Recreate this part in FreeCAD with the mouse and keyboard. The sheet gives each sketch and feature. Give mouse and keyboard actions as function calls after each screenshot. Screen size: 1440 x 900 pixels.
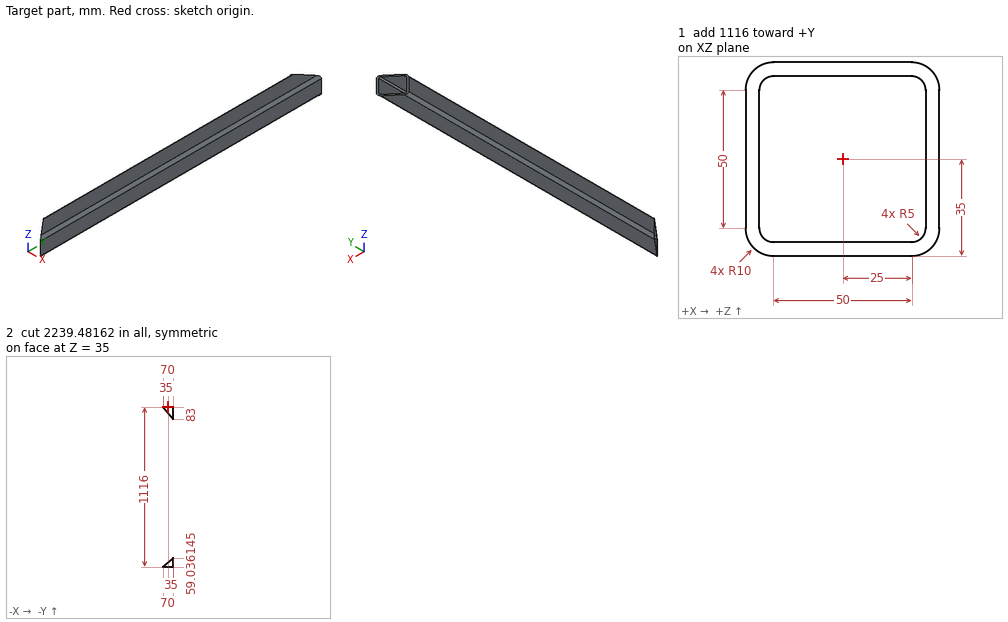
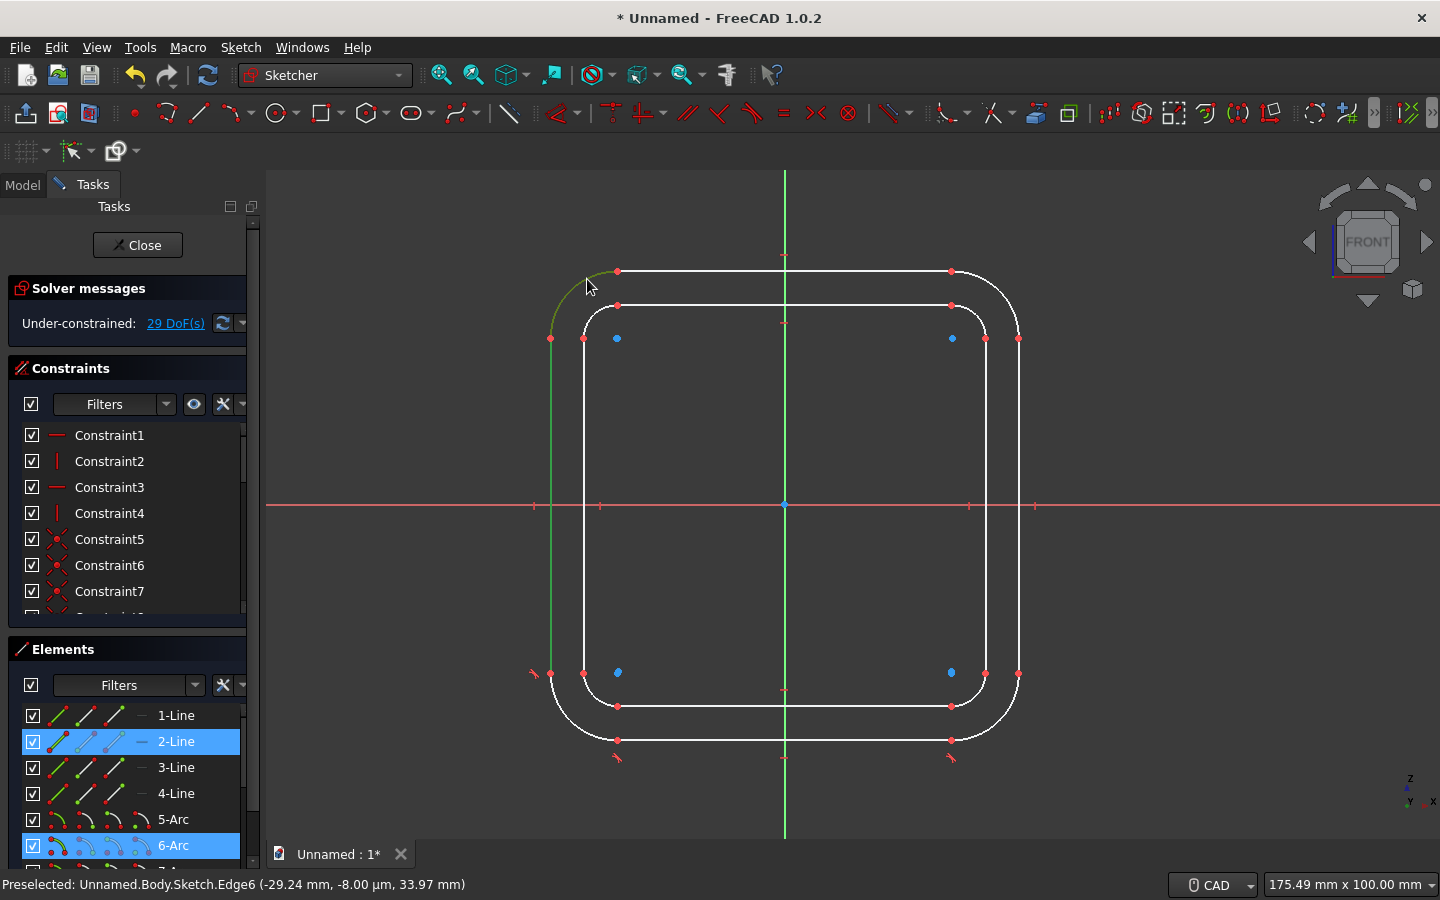
key(t)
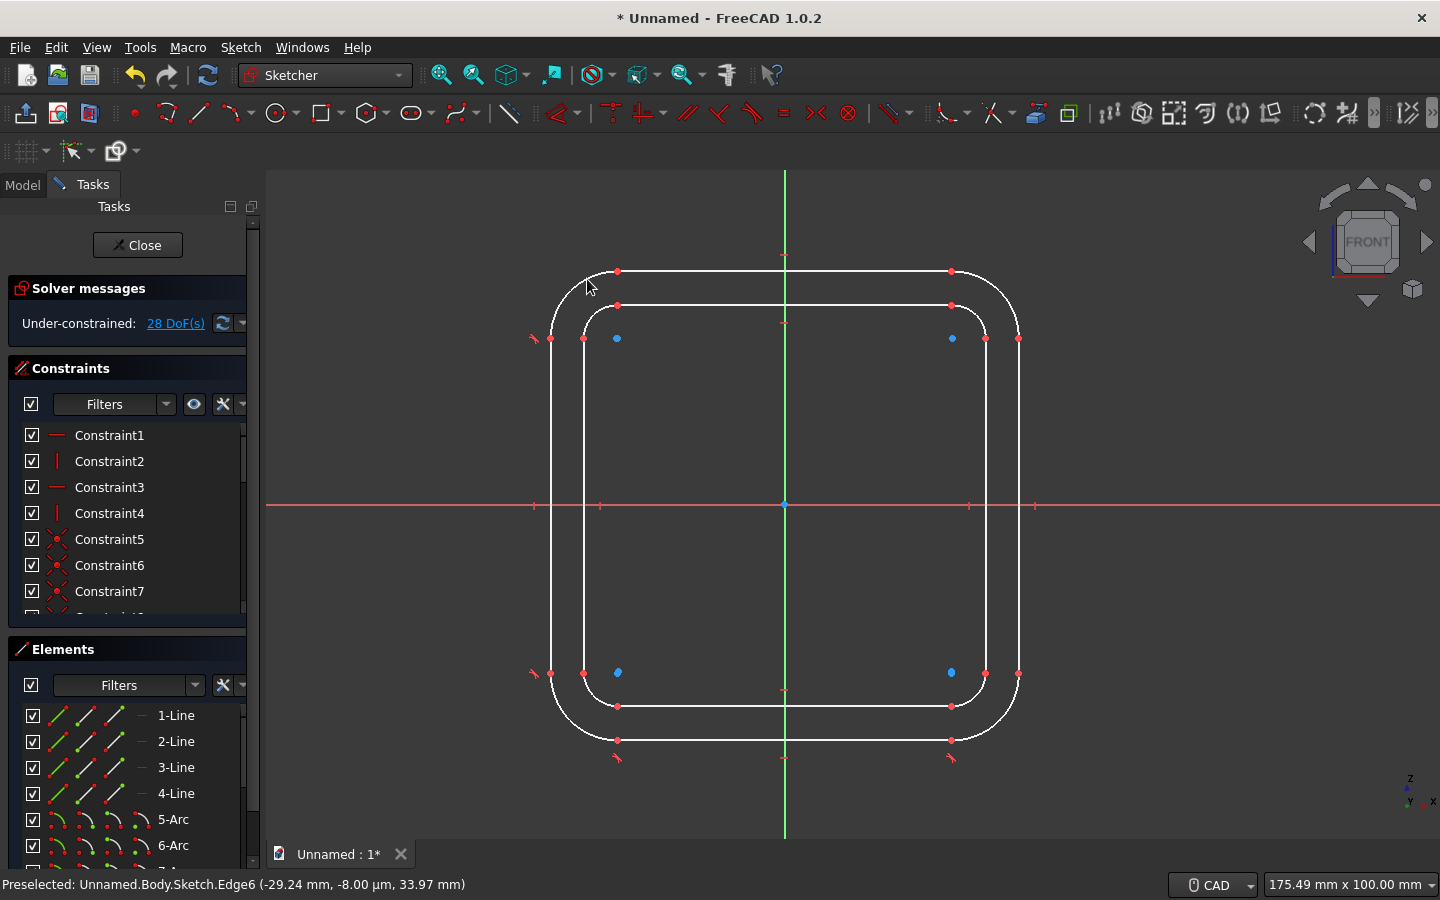
click(718, 271)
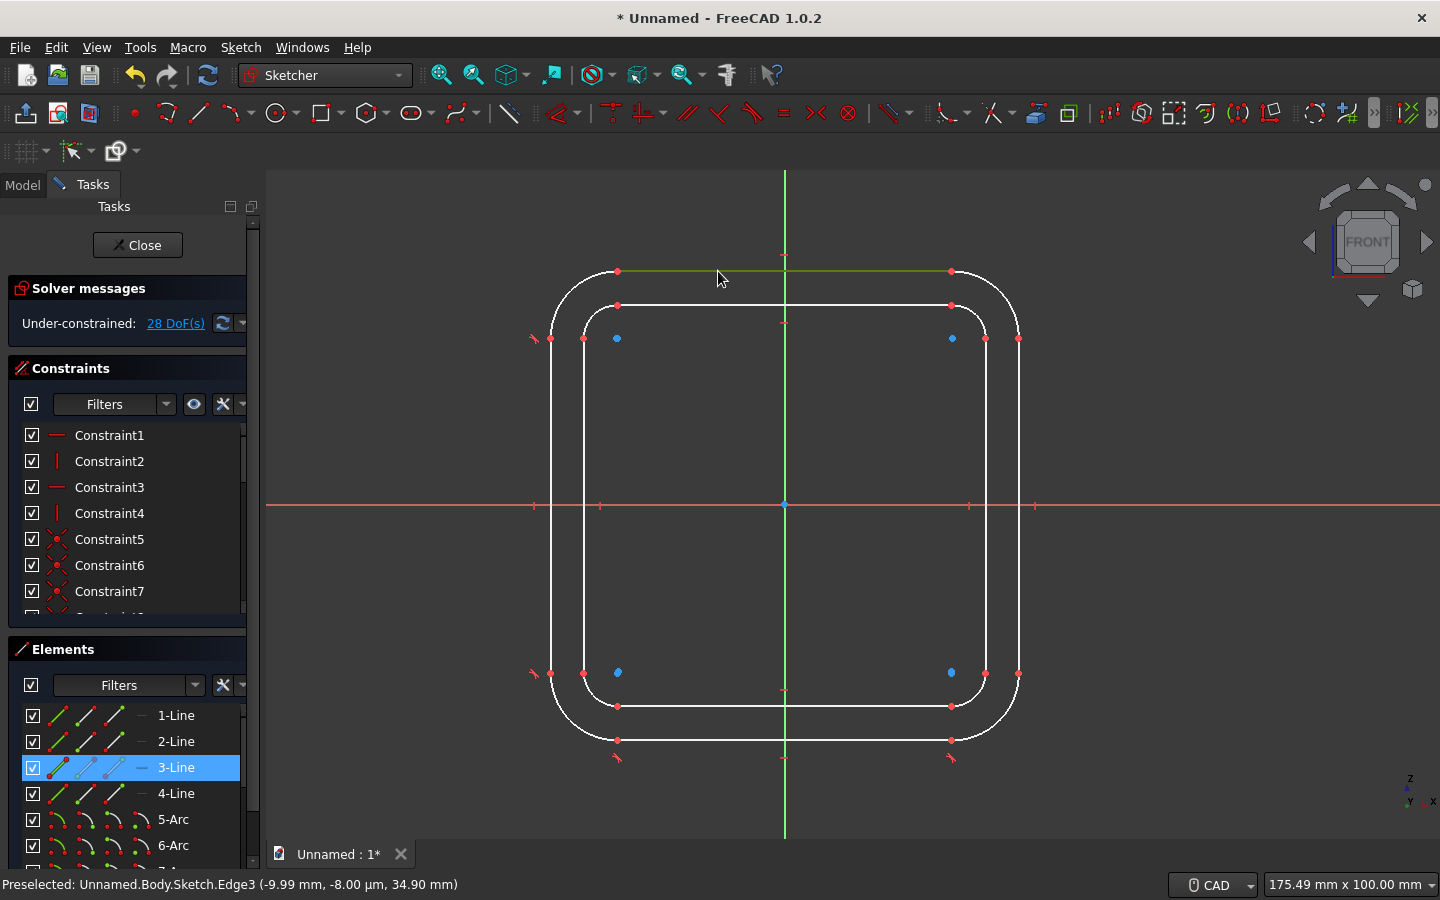
click(587, 279)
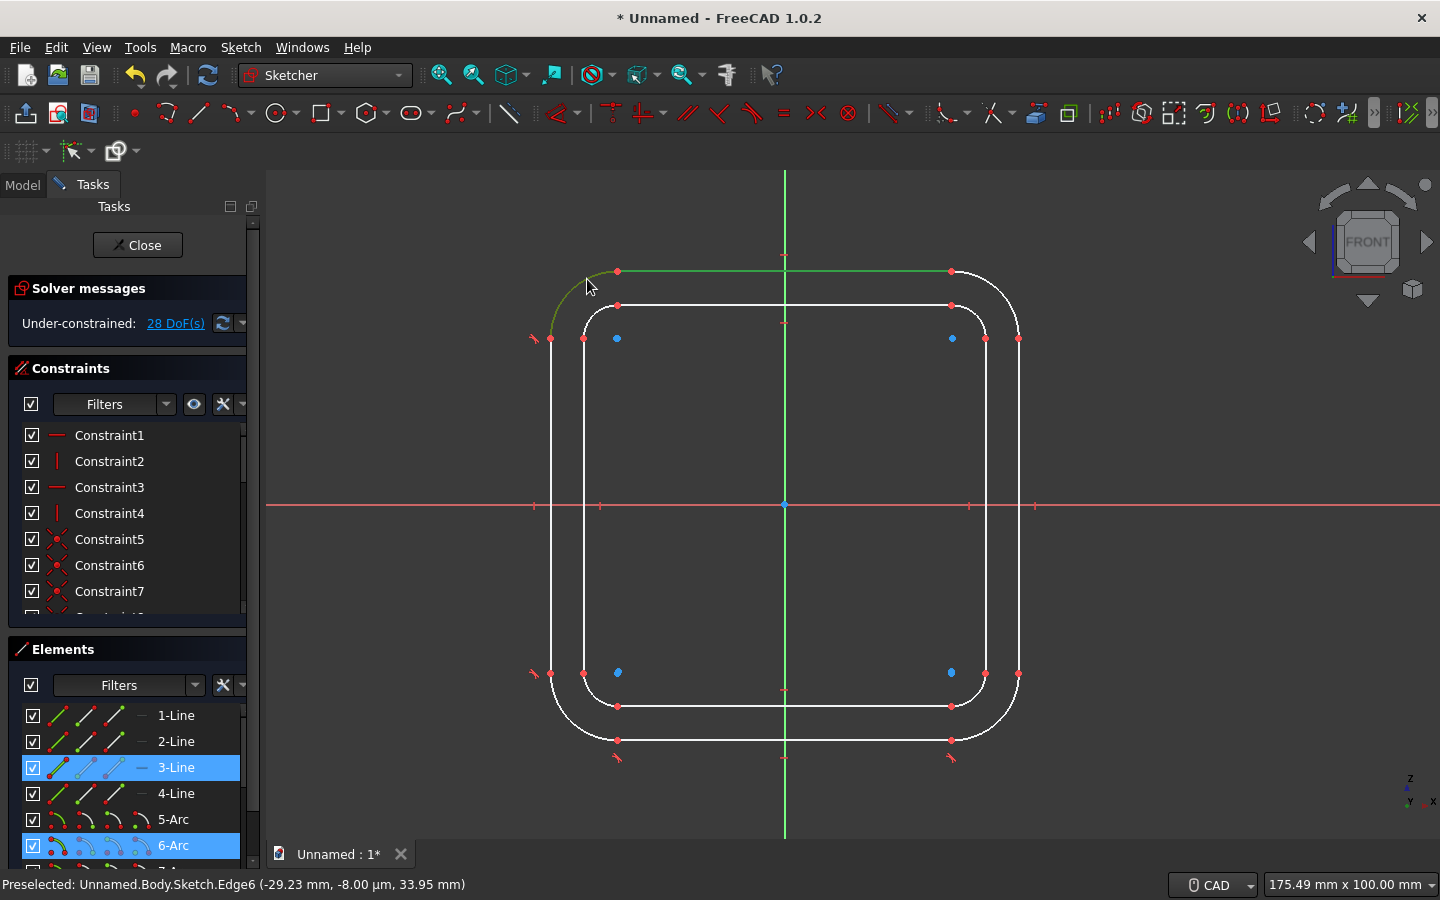
key(t)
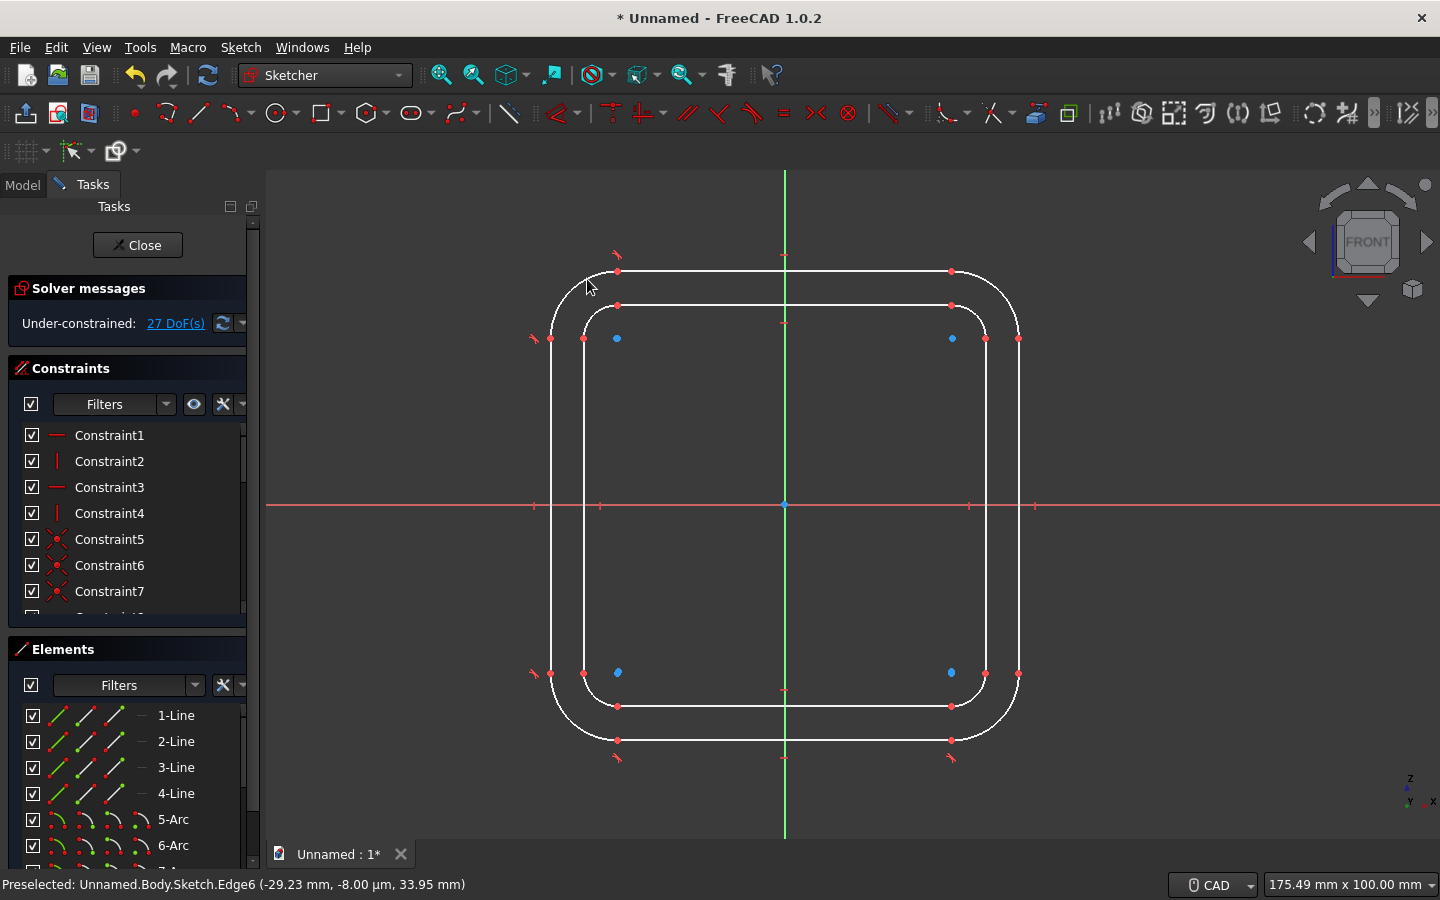
click(718, 271)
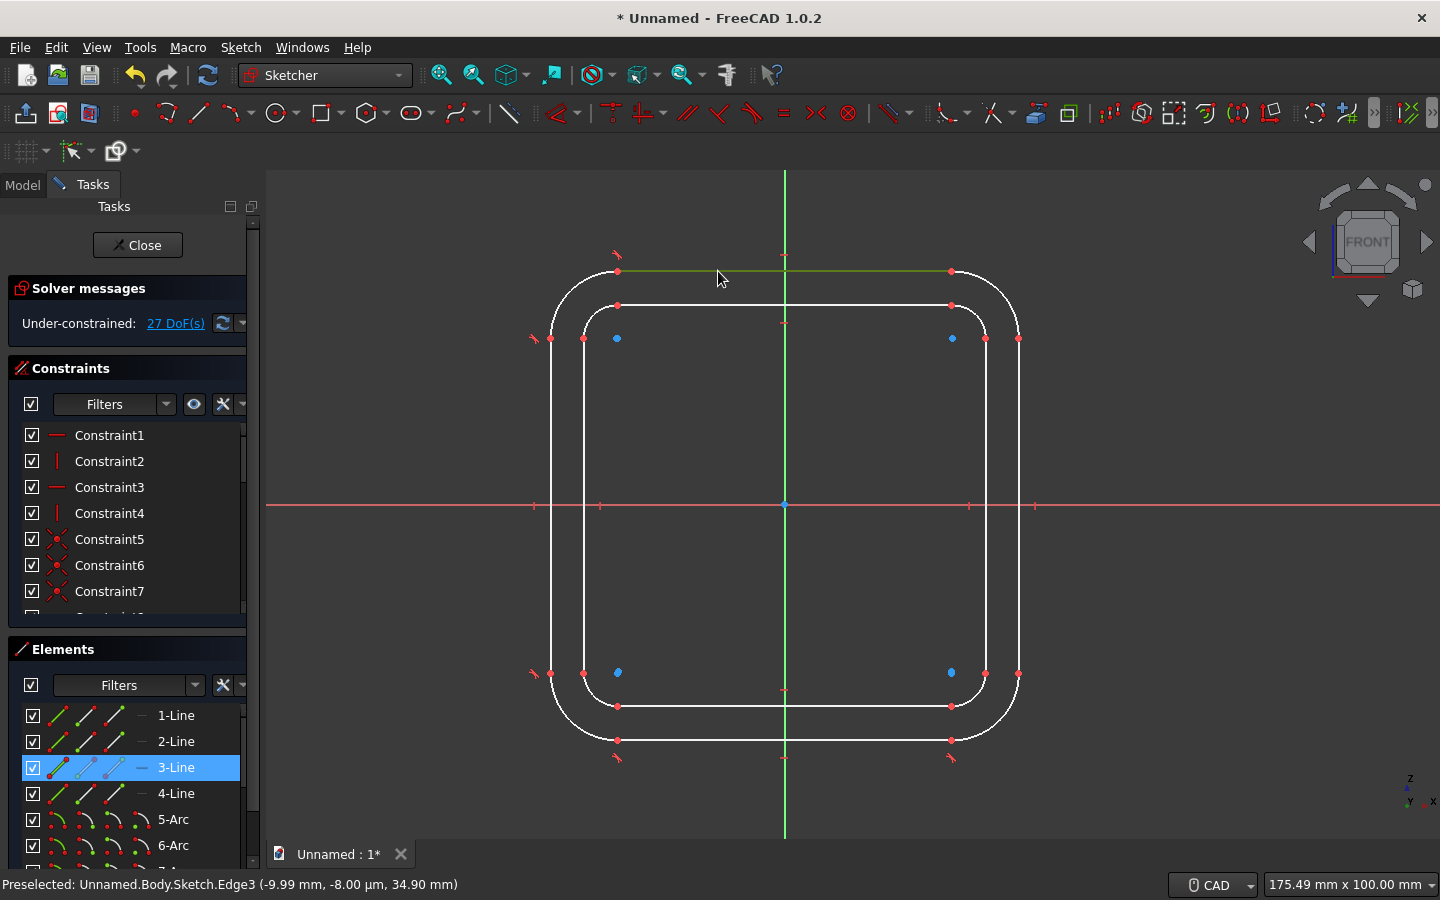
click(1012, 308)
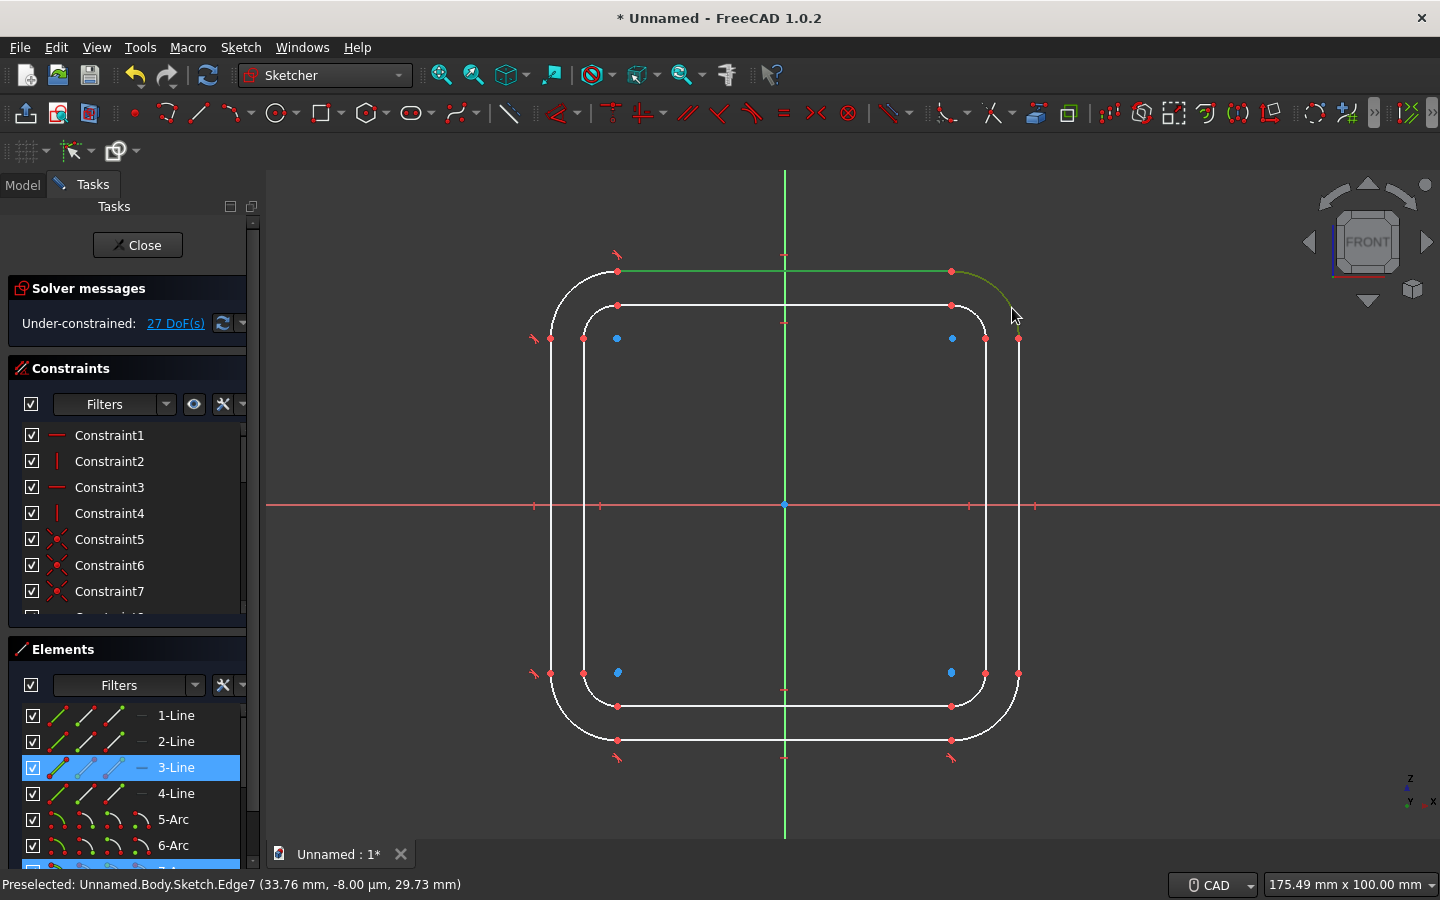
click(752, 114)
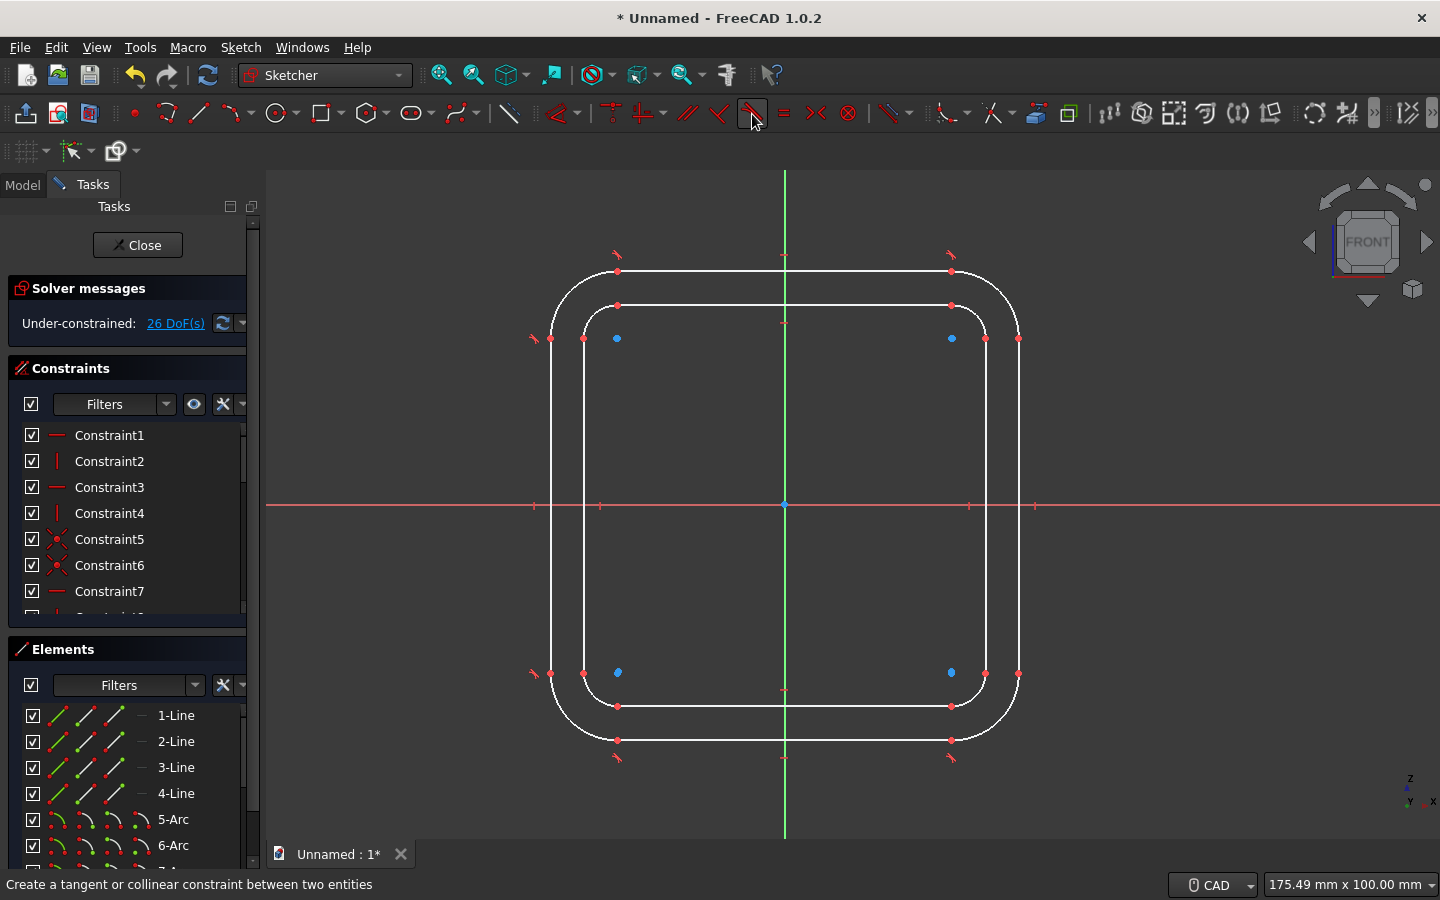
click(1019, 439)